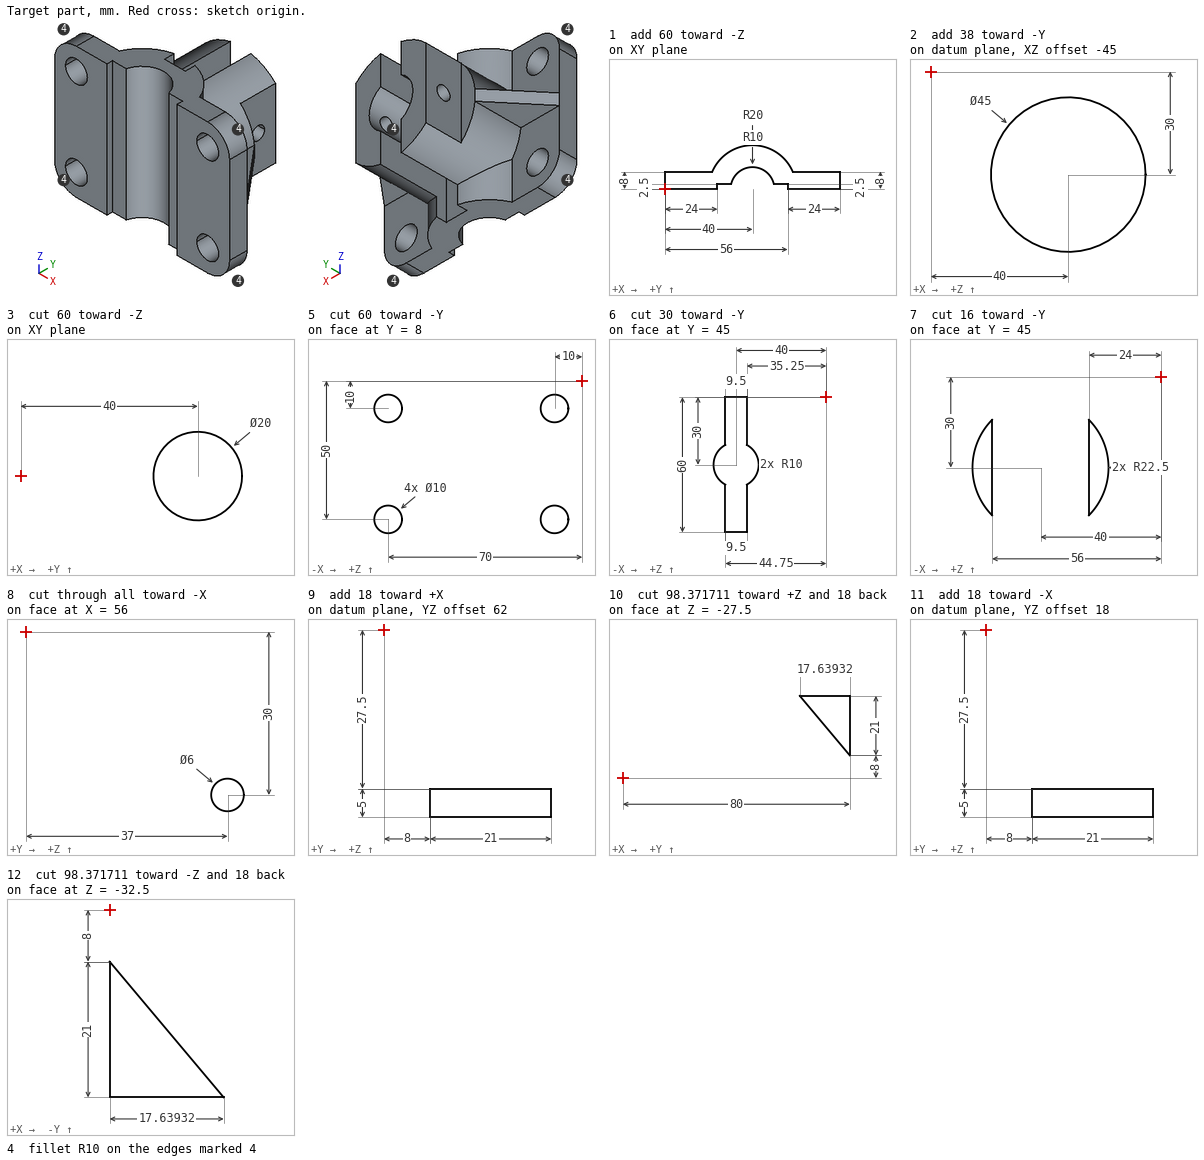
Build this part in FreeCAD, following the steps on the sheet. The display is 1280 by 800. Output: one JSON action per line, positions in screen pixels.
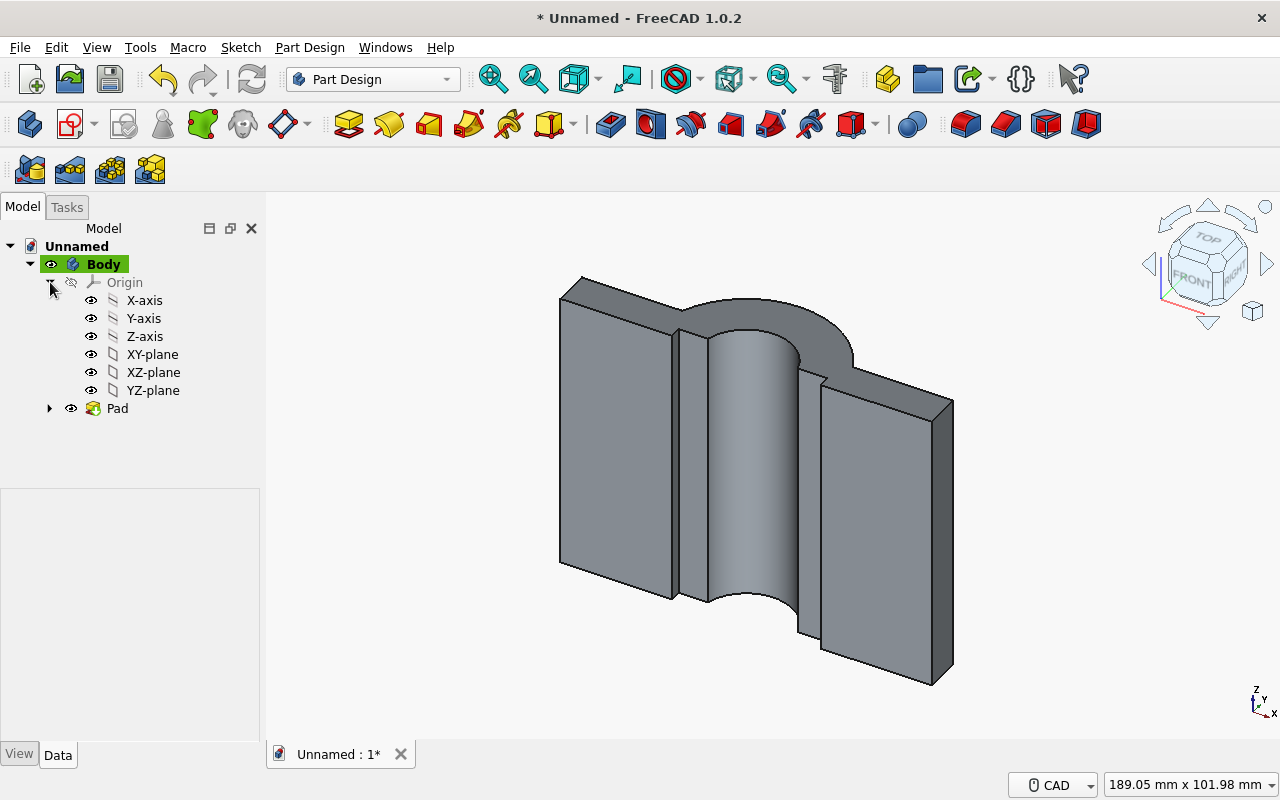
{"action": "left_click", "coordinate": [136, 372]}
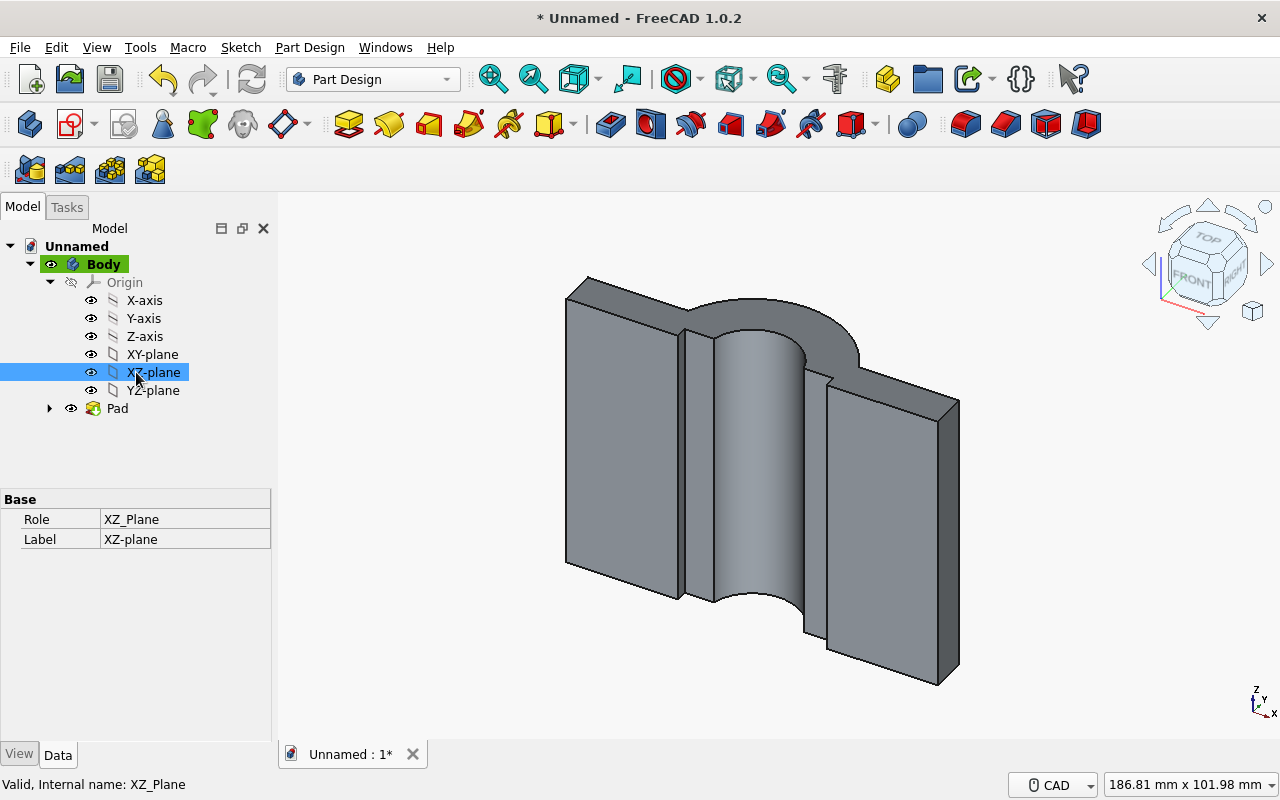
{"action": "left_click", "coordinate": [284, 124]}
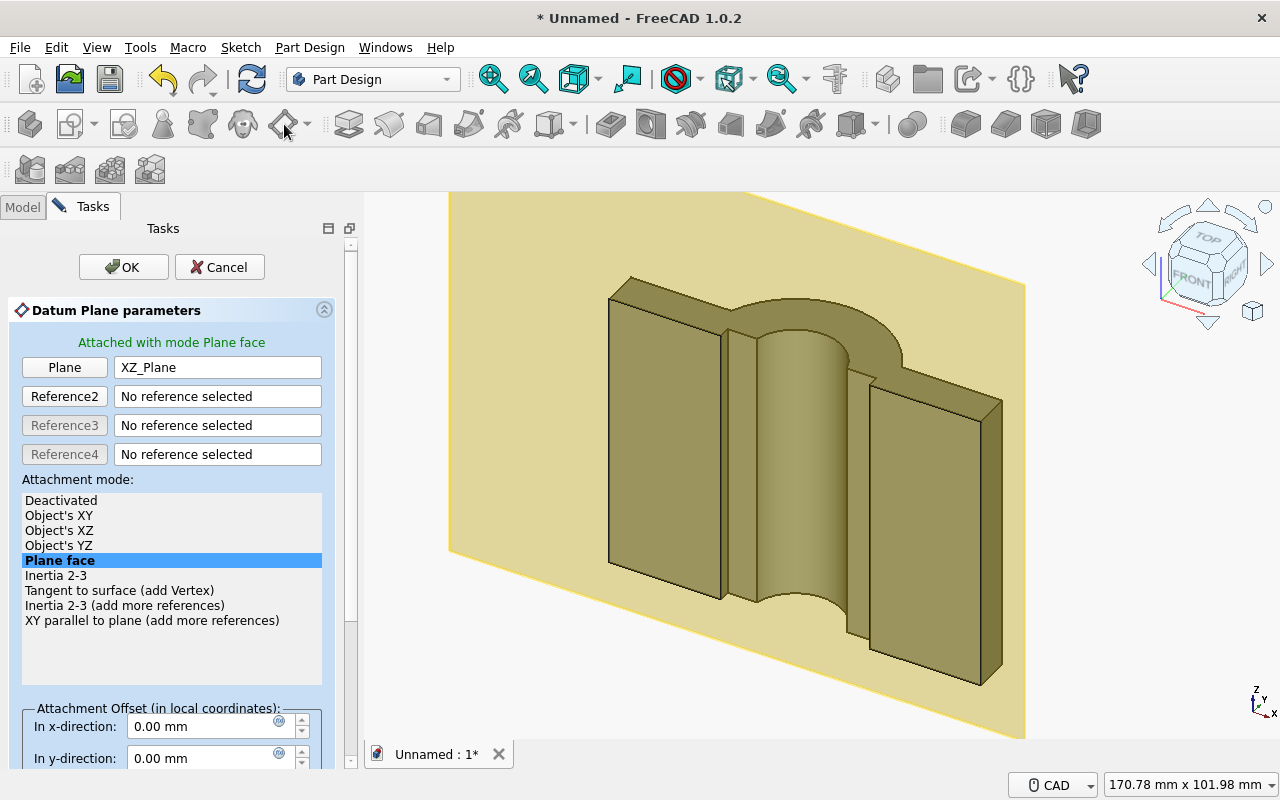
{"action": "scroll", "coordinate": [351, 503], "scroll_direction": "down", "scroll_amount": 2}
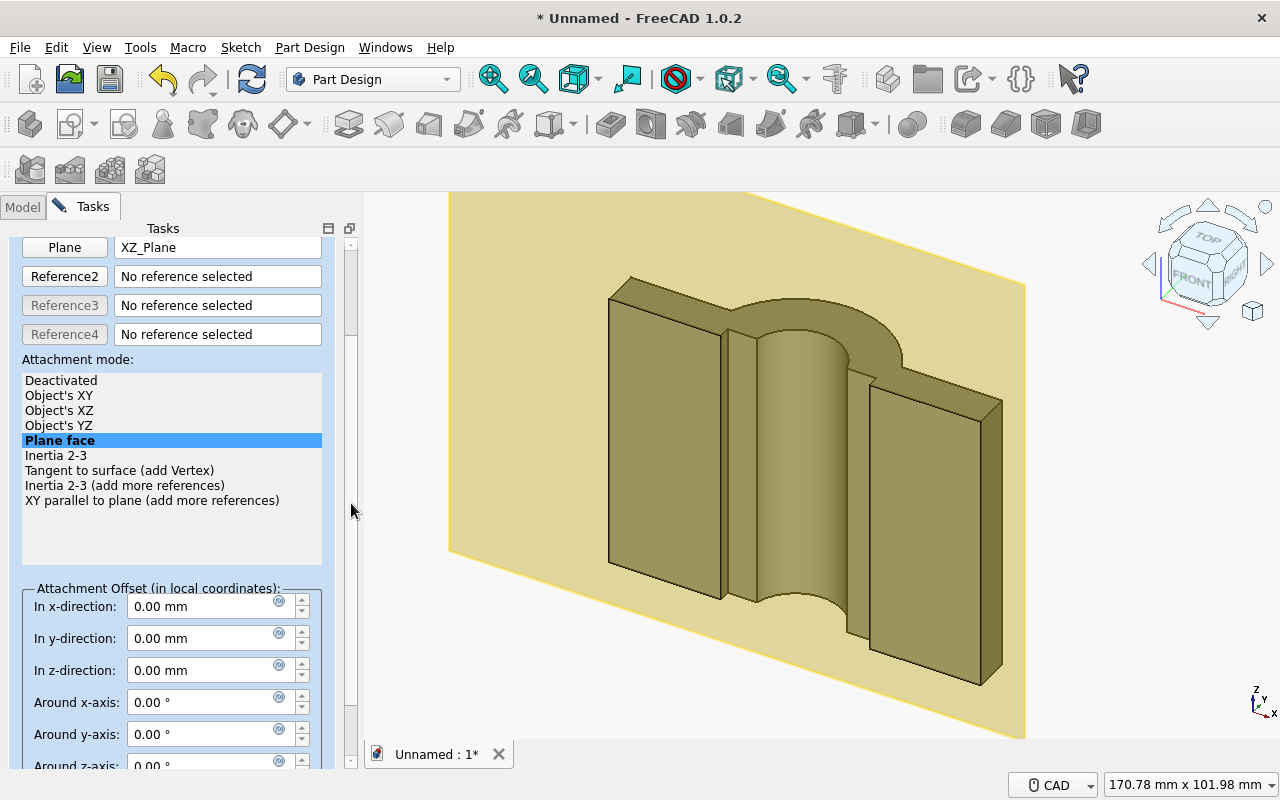
{"action": "triple_click", "coordinate": [210, 670]}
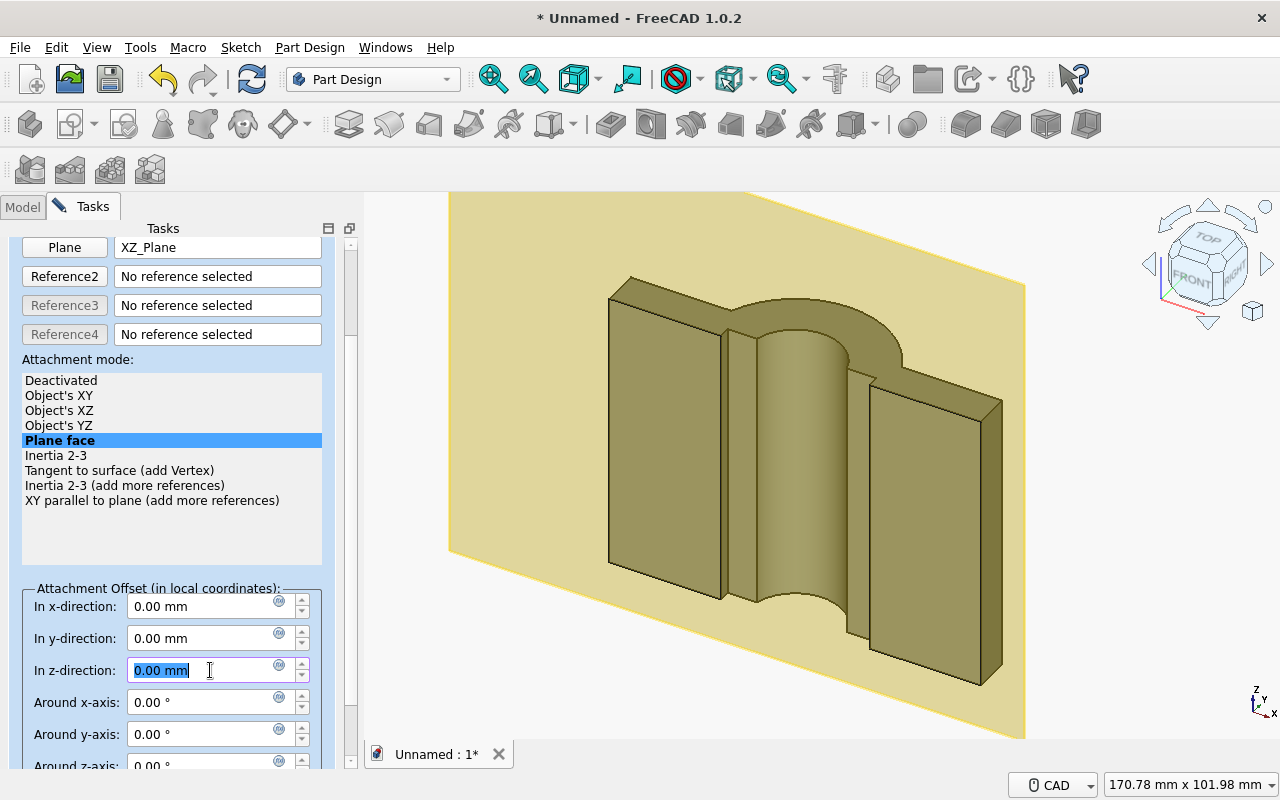
{"action": "type", "text": "-45"}
{"action": "key", "text": "Tab"}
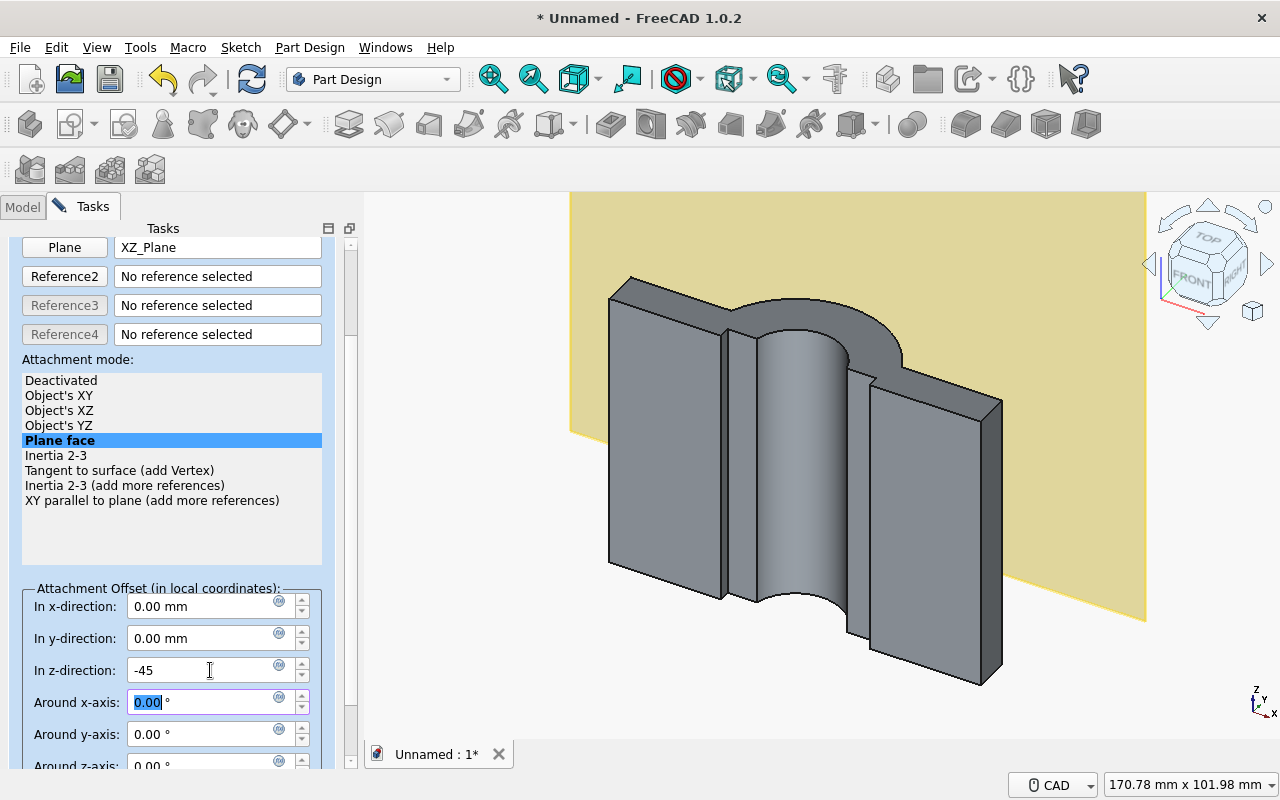
{"action": "scroll", "coordinate": [351, 503], "scroll_direction": "up", "scroll_amount": 3}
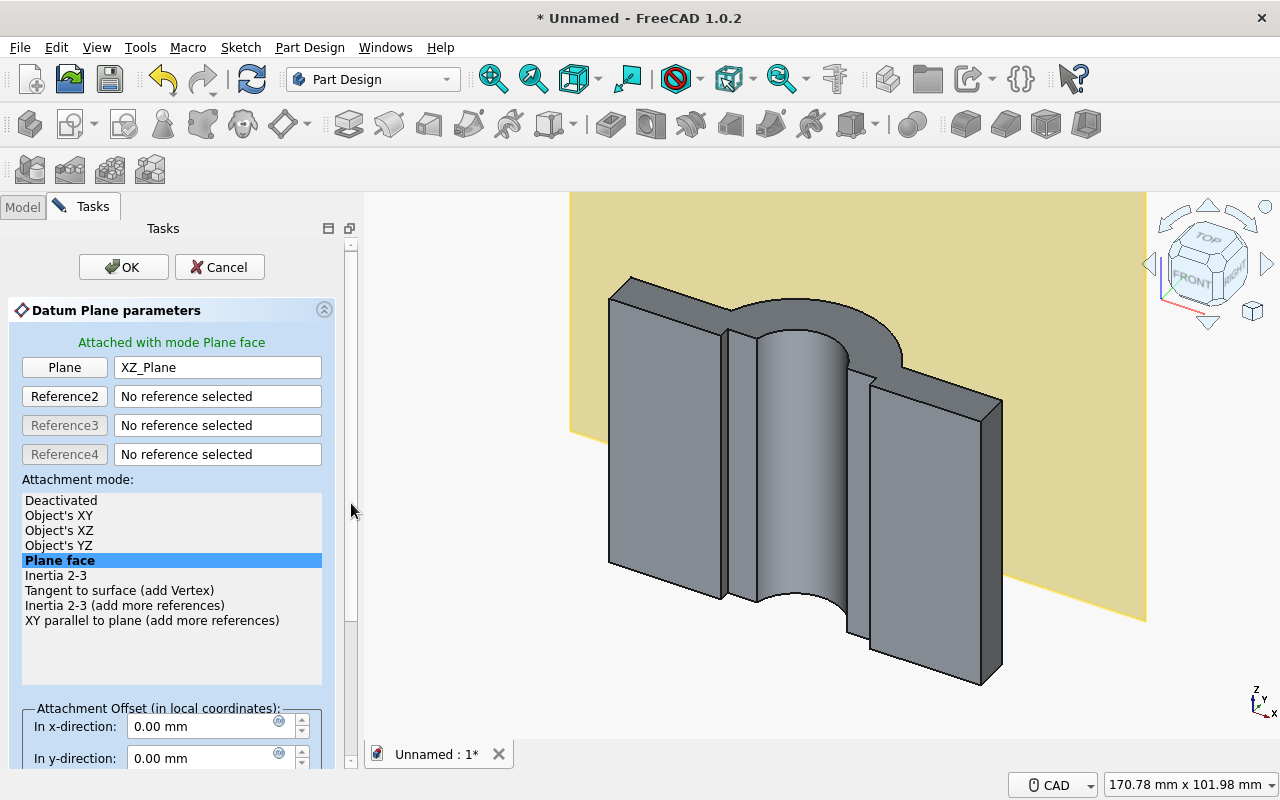
{"action": "left_click", "coordinate": [124, 267]}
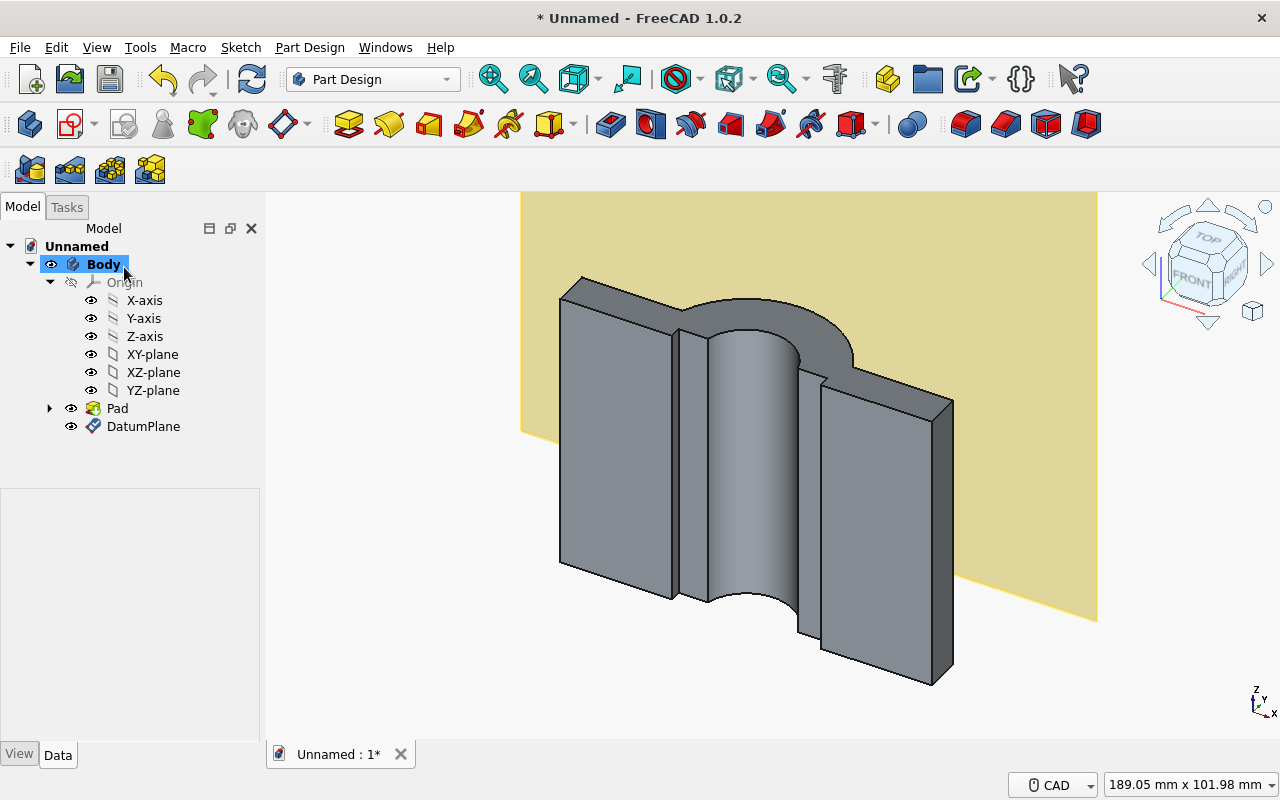
{"action": "left_click", "coordinate": [116, 426]}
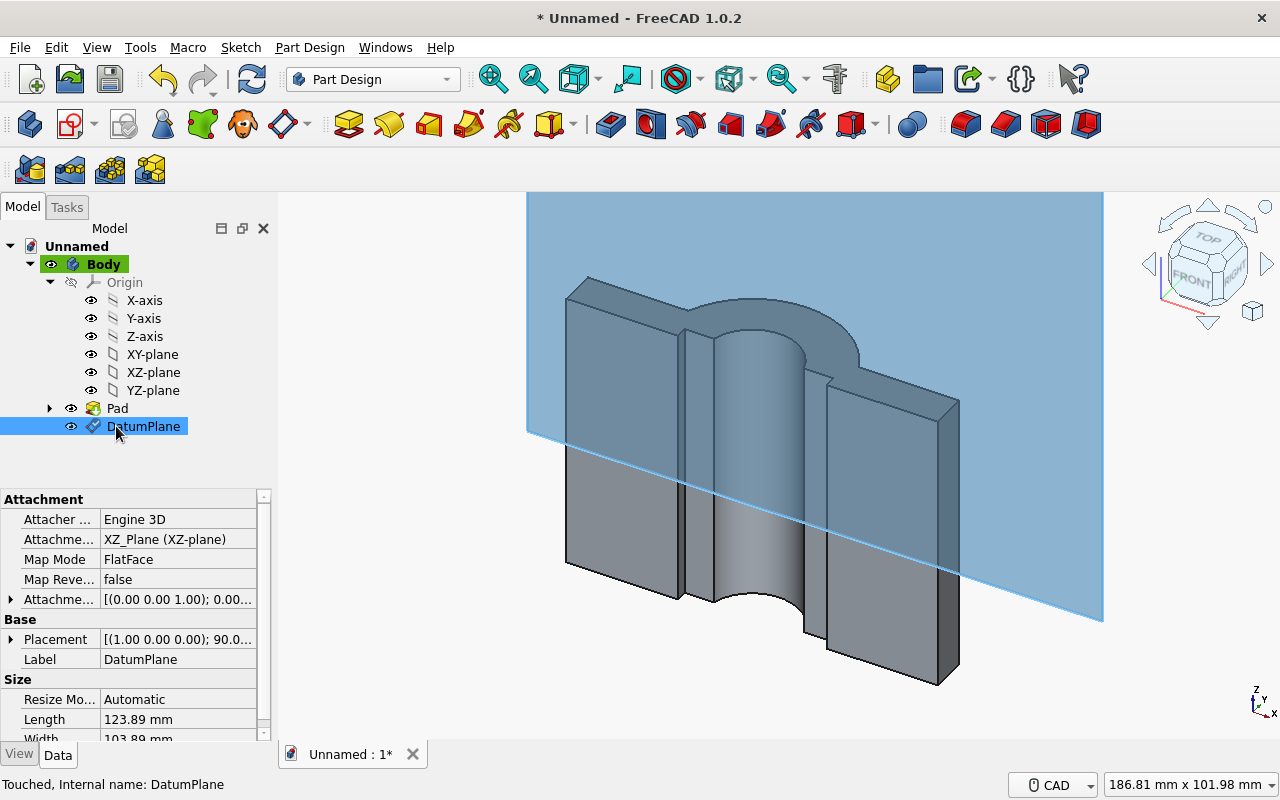
{"action": "left_click", "coordinate": [70, 124]}